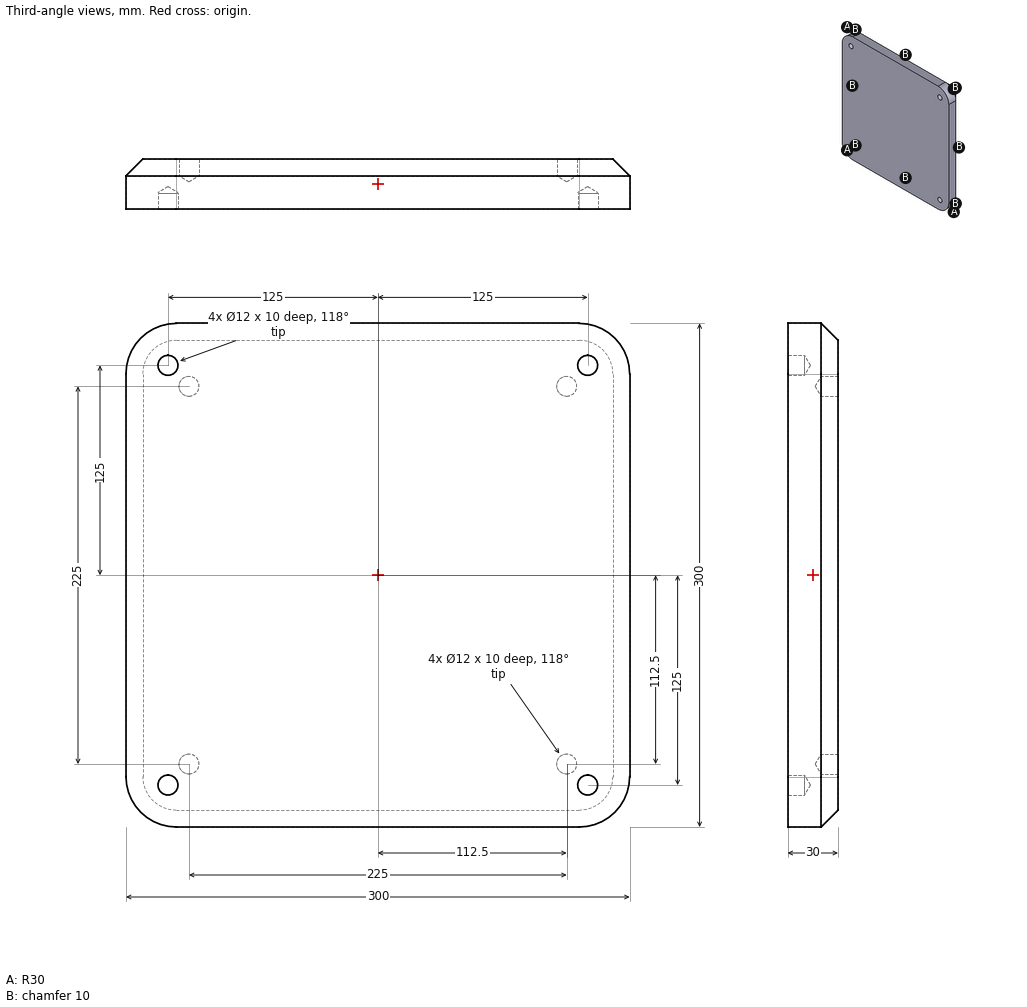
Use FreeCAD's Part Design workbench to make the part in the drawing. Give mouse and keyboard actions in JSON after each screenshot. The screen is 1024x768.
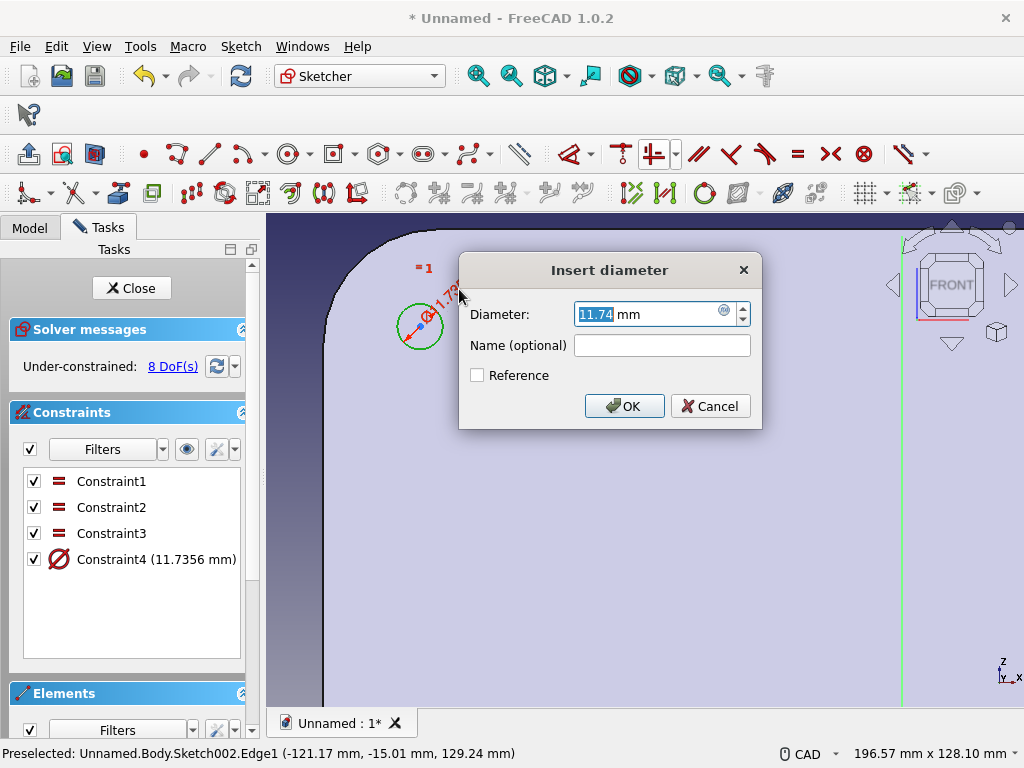
{"action": "type", "text": "12"}
{"action": "key", "text": "Return"}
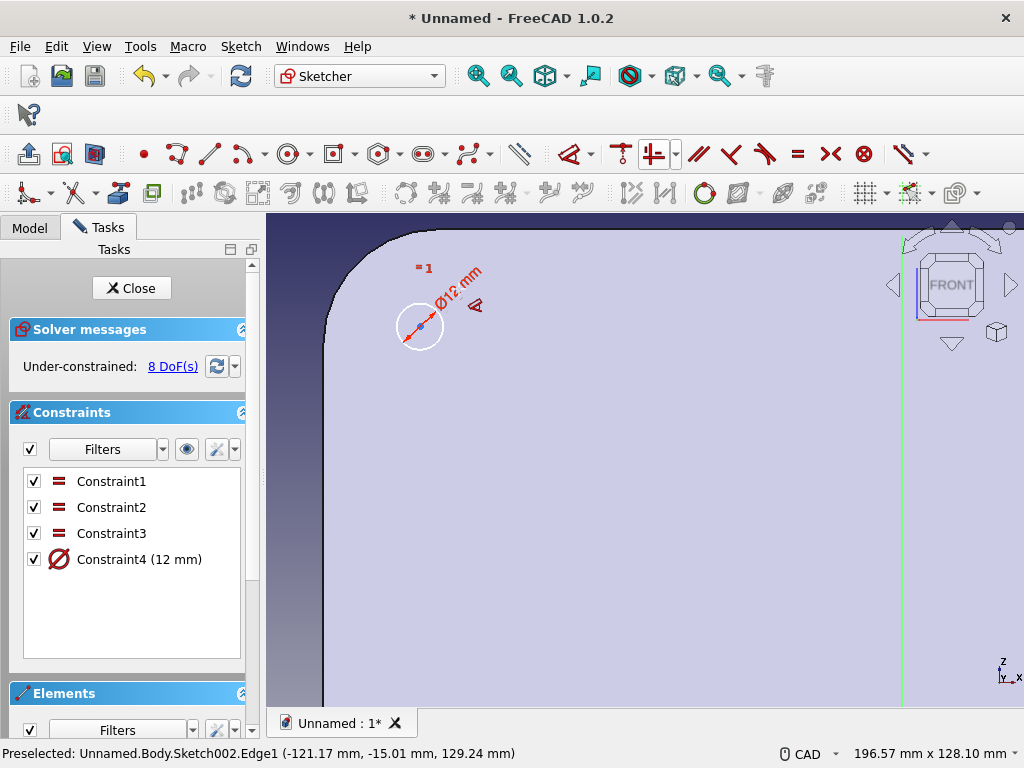
{"action": "left_click", "coordinate": [420, 327]}
{"action": "left_click", "coordinate": [640, 293]}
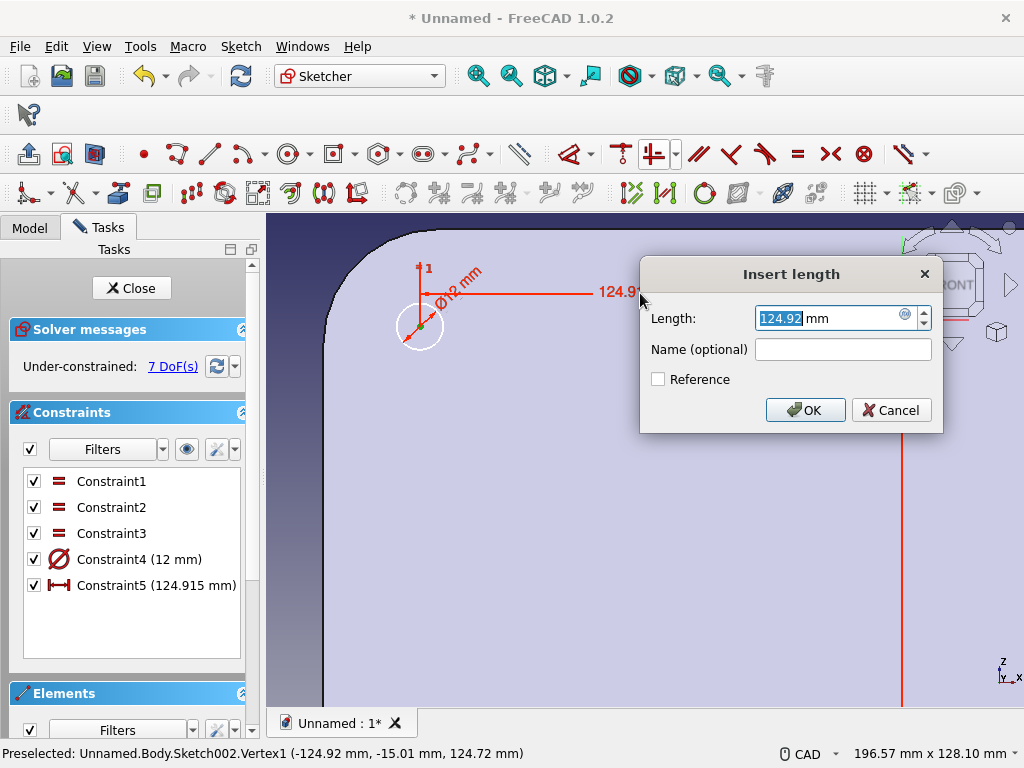
{"action": "type", "text": "125"}
{"action": "key", "text": "Return"}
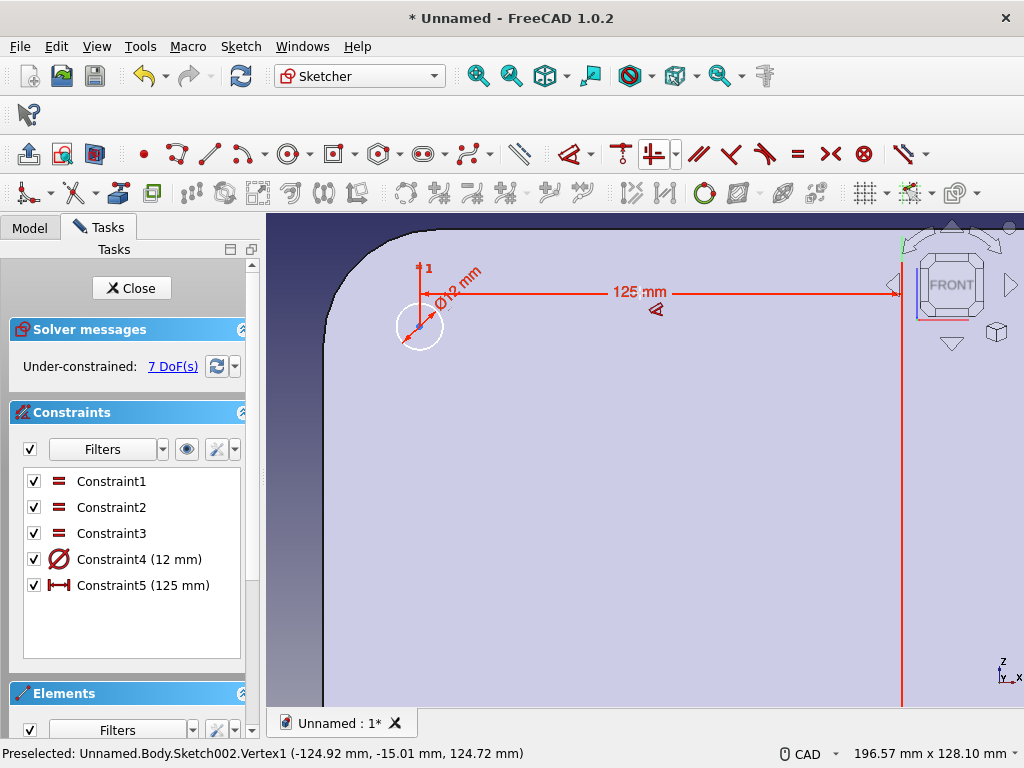
{"action": "left_click", "coordinate": [420, 327]}
{"action": "left_click", "coordinate": [386, 503]}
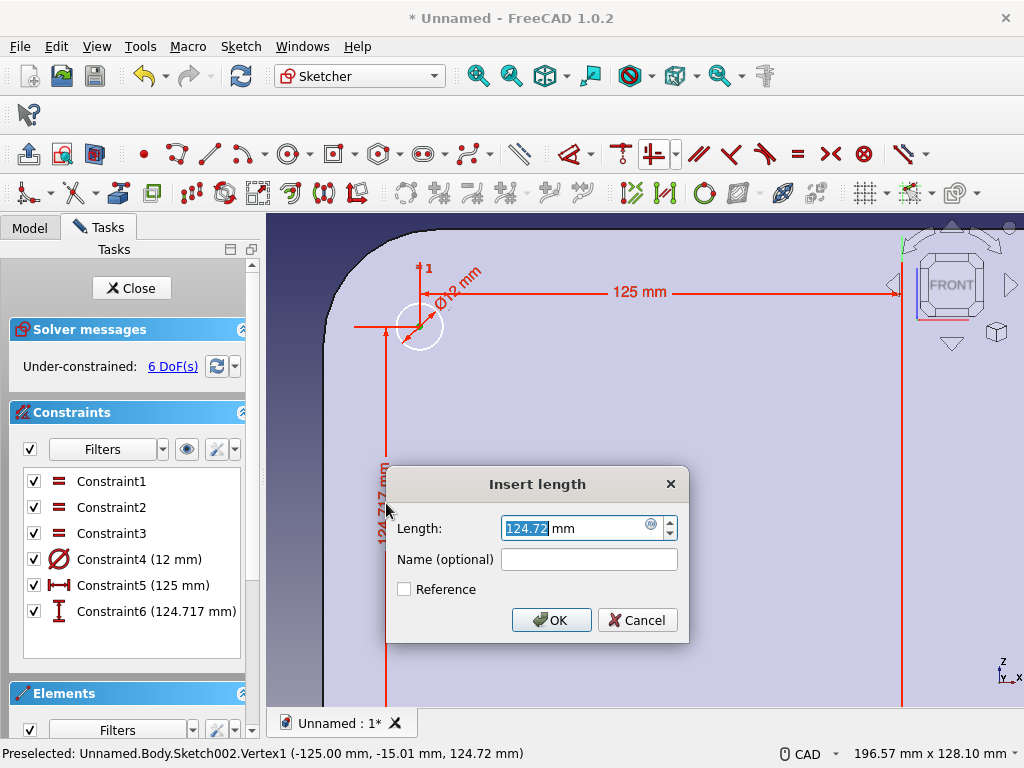
{"action": "type", "text": "125"}
{"action": "key", "text": "Return"}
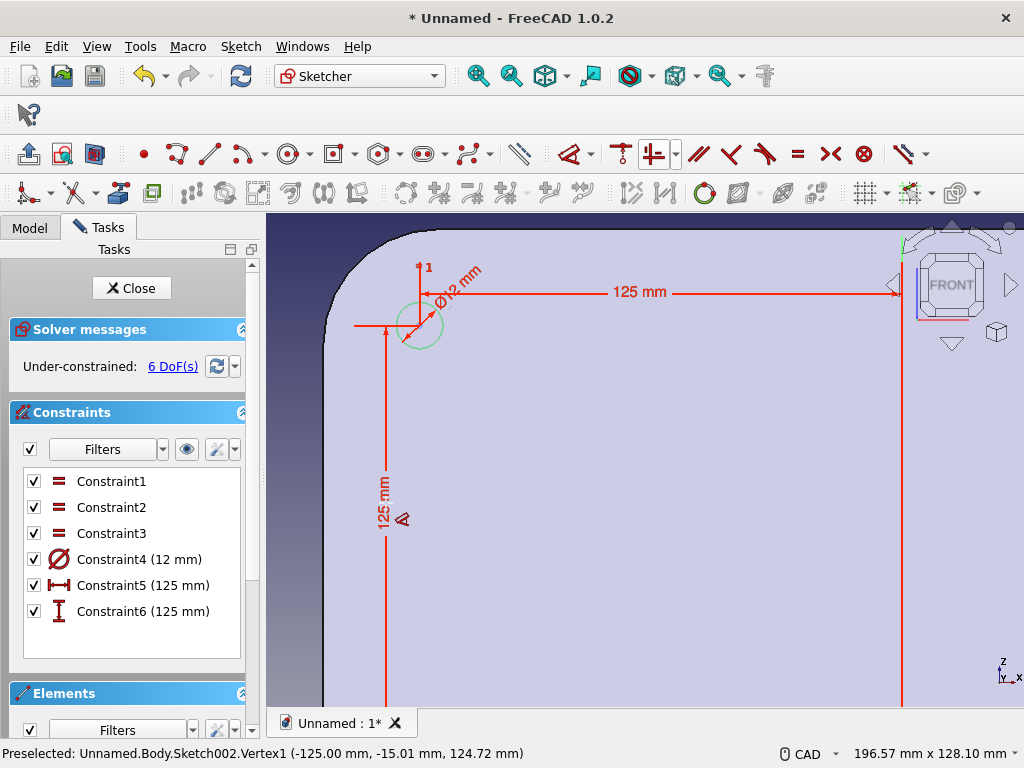
{"action": "scroll", "coordinate": [436, 310], "scroll_direction": "down", "scroll_amount": 6}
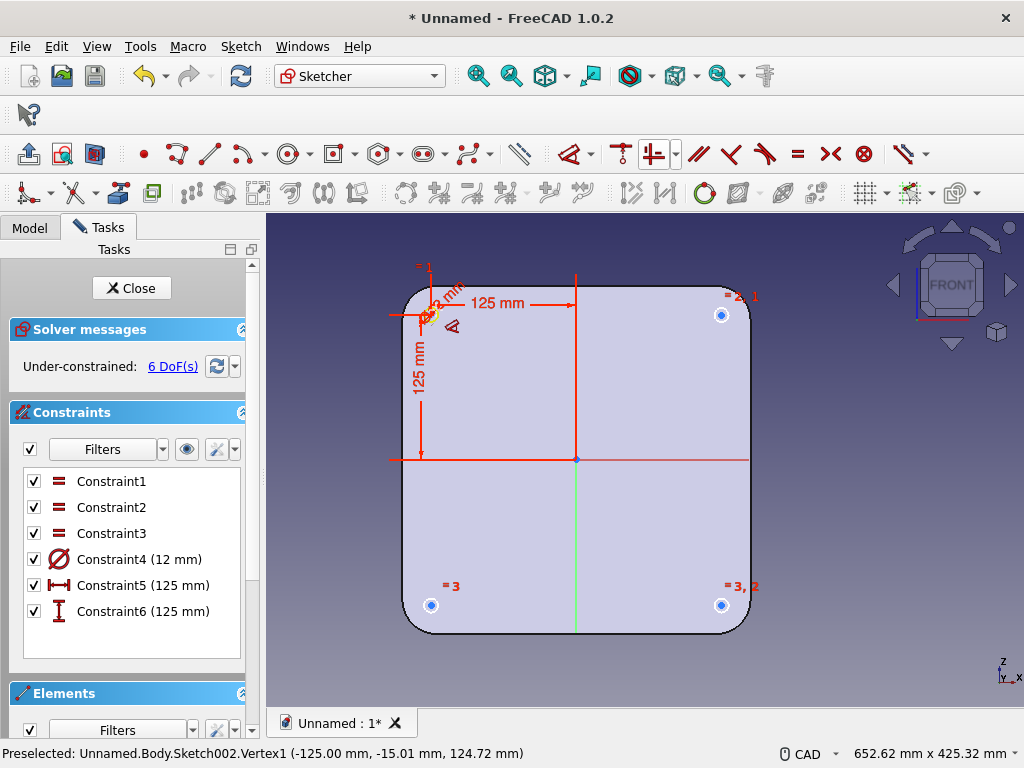
{"action": "left_click", "coordinate": [722, 315]}
{"action": "left_click", "coordinate": [649, 281]}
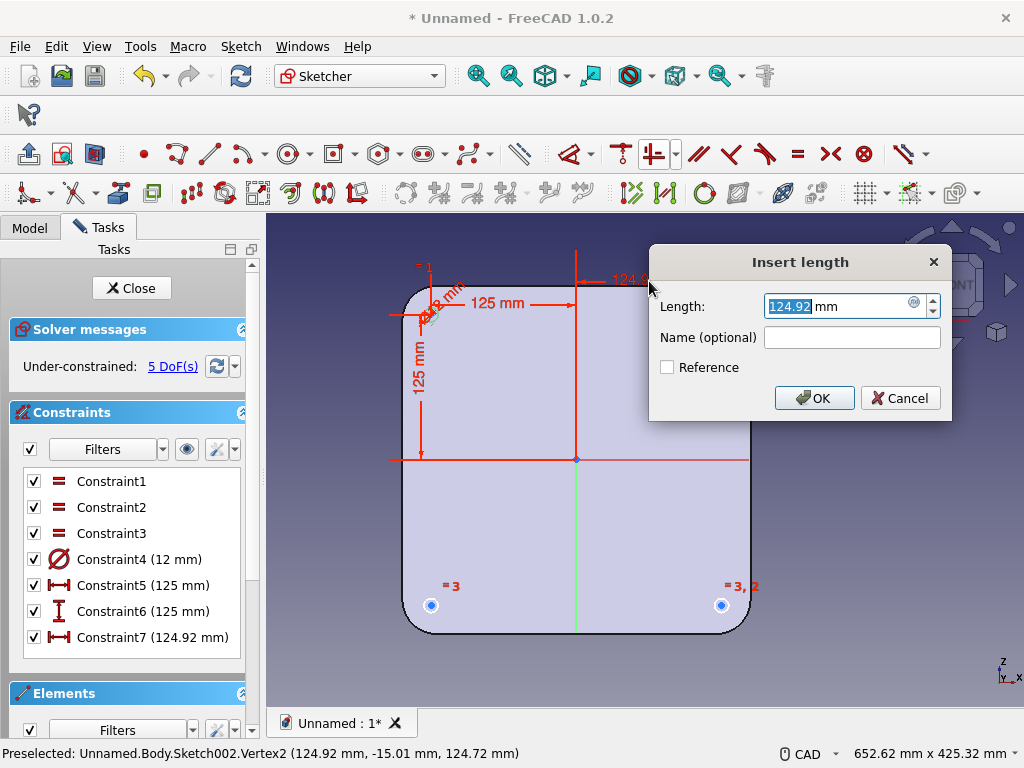
{"action": "type", "text": "125"}
{"action": "key", "text": "Return"}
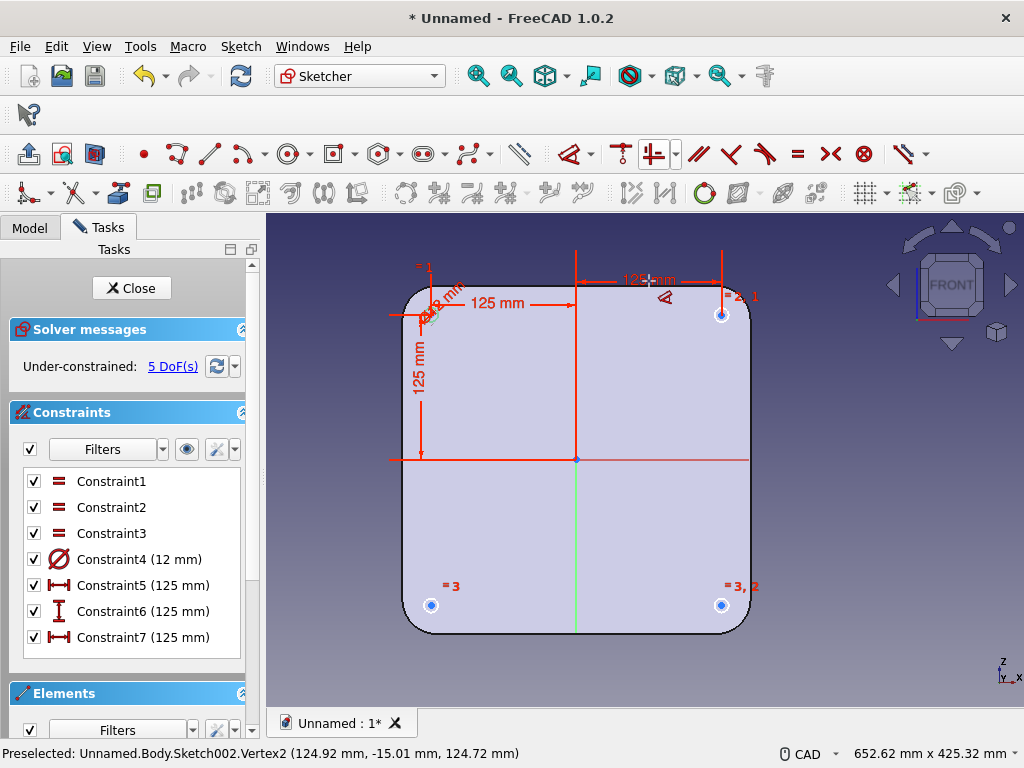
{"action": "left_click", "coordinate": [722, 315]}
{"action": "left_click", "coordinate": [756, 388]}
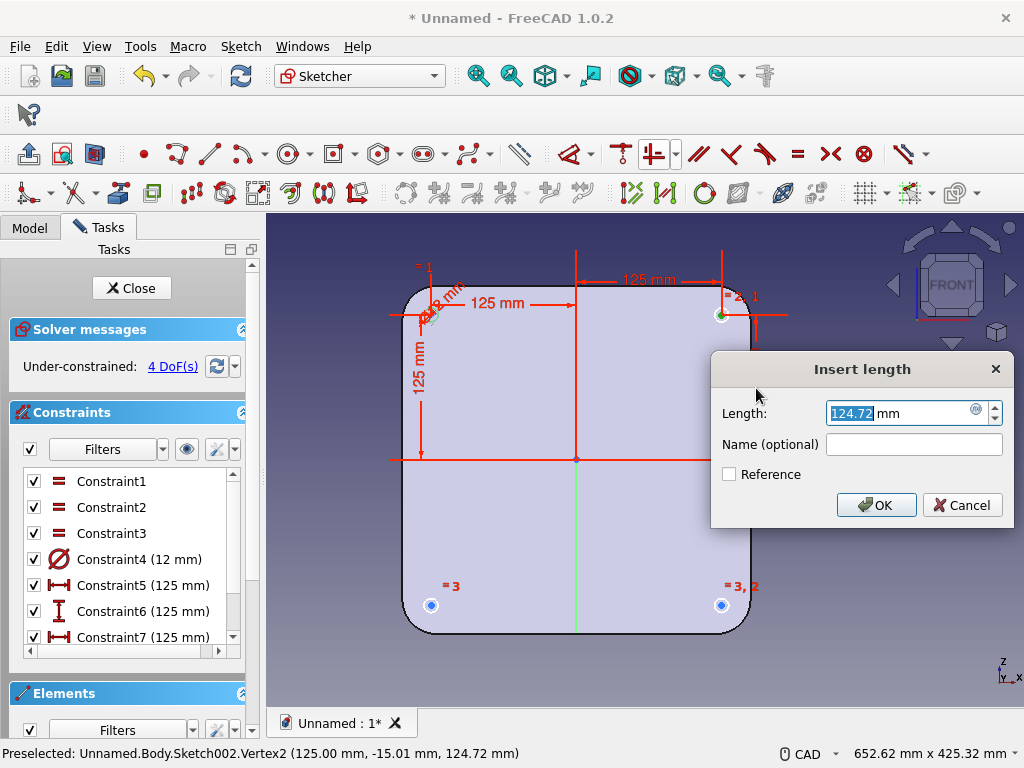
{"action": "type", "text": "125"}
{"action": "key", "text": "Return"}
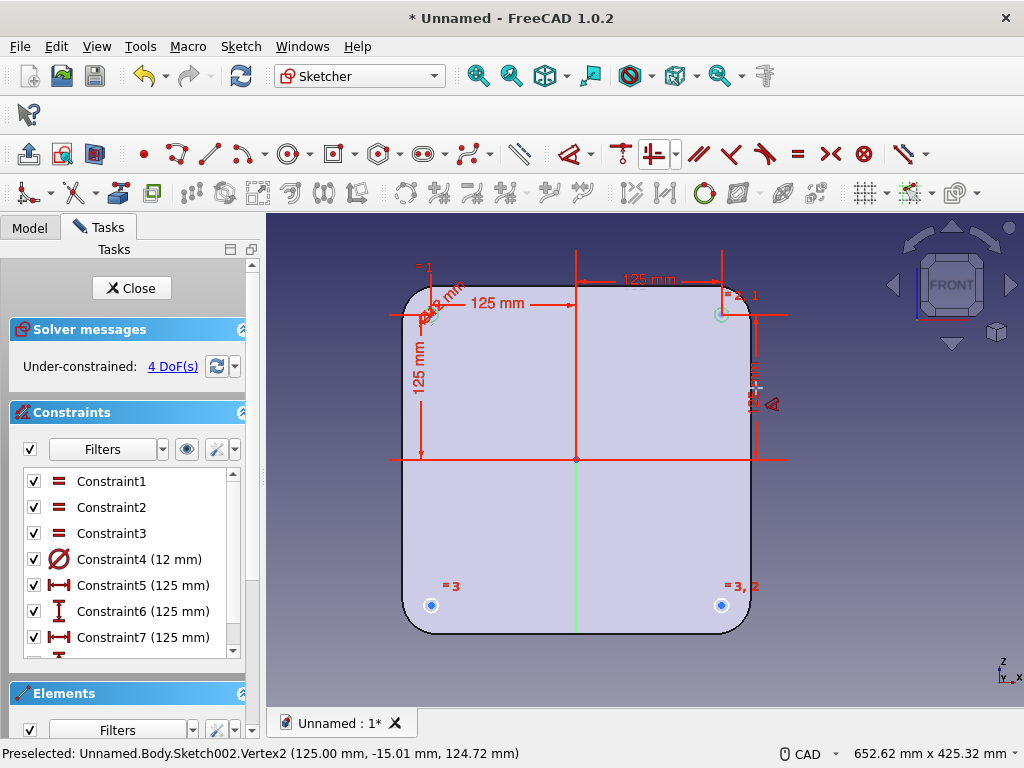
{"action": "left_click", "coordinate": [722, 606]}
{"action": "left_click", "coordinate": [649, 640]}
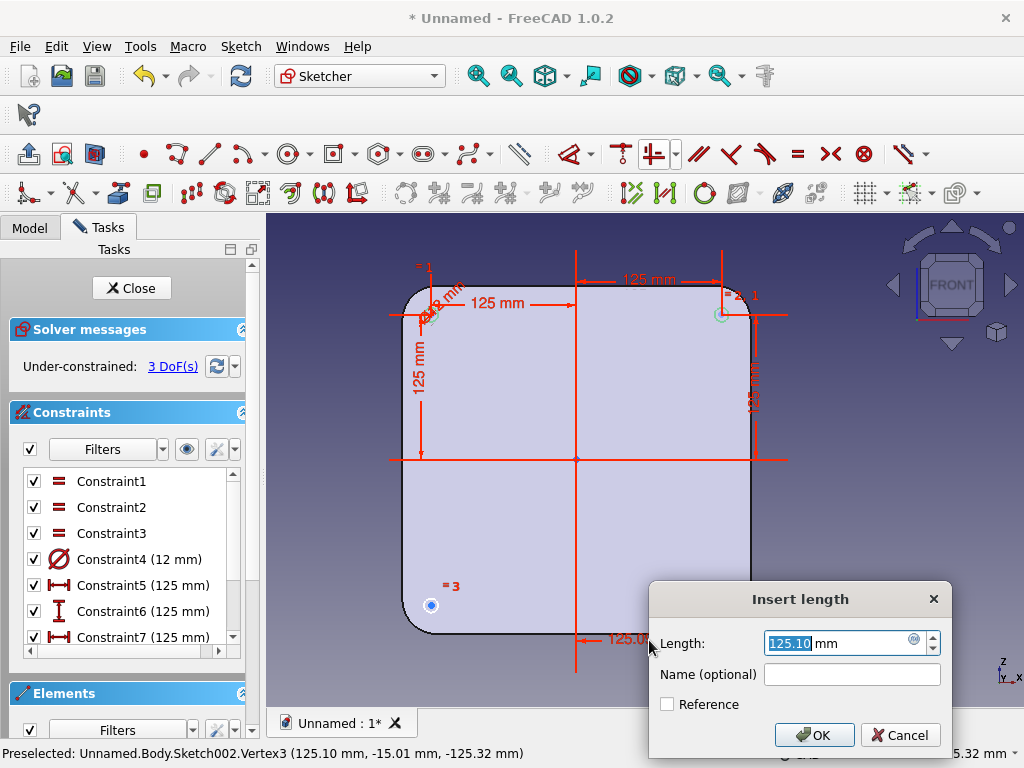
{"action": "type", "text": "125"}
{"action": "key", "text": "Return"}